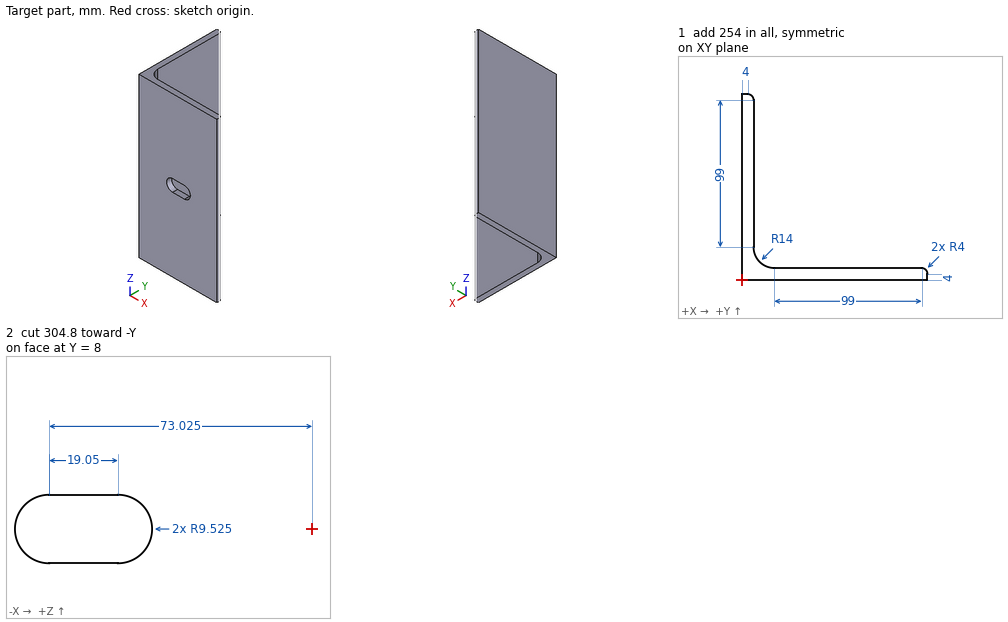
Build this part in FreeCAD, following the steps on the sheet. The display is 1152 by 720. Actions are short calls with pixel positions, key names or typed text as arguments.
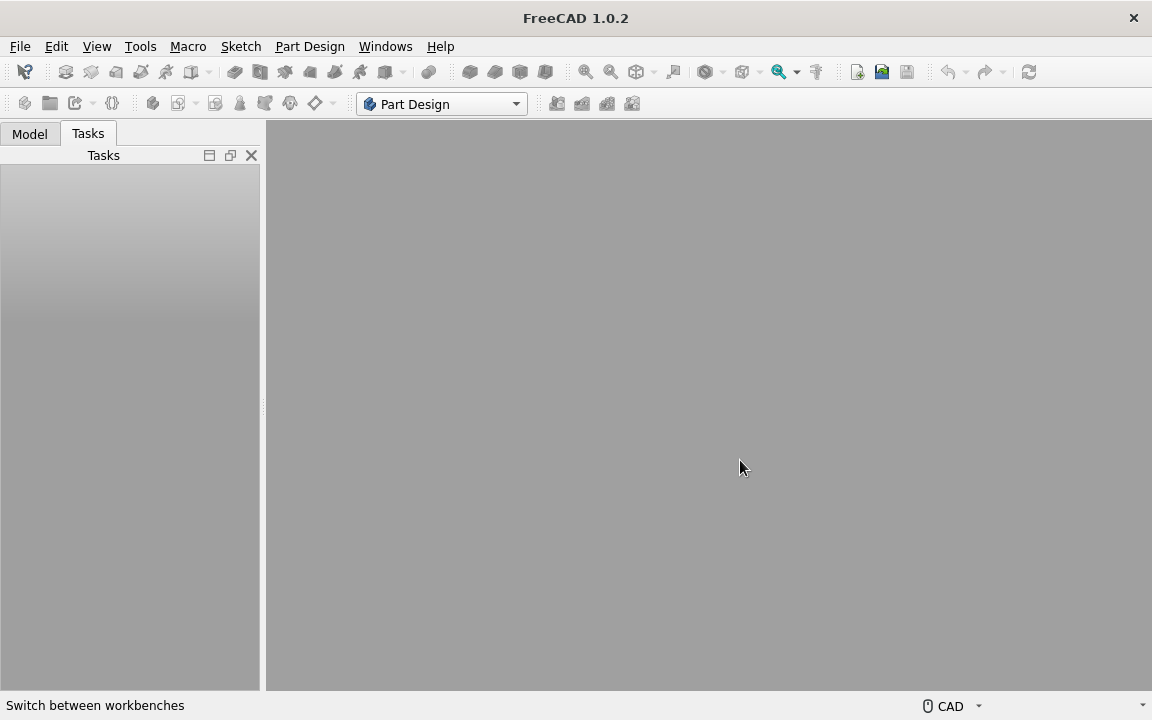
key(ctrl+n)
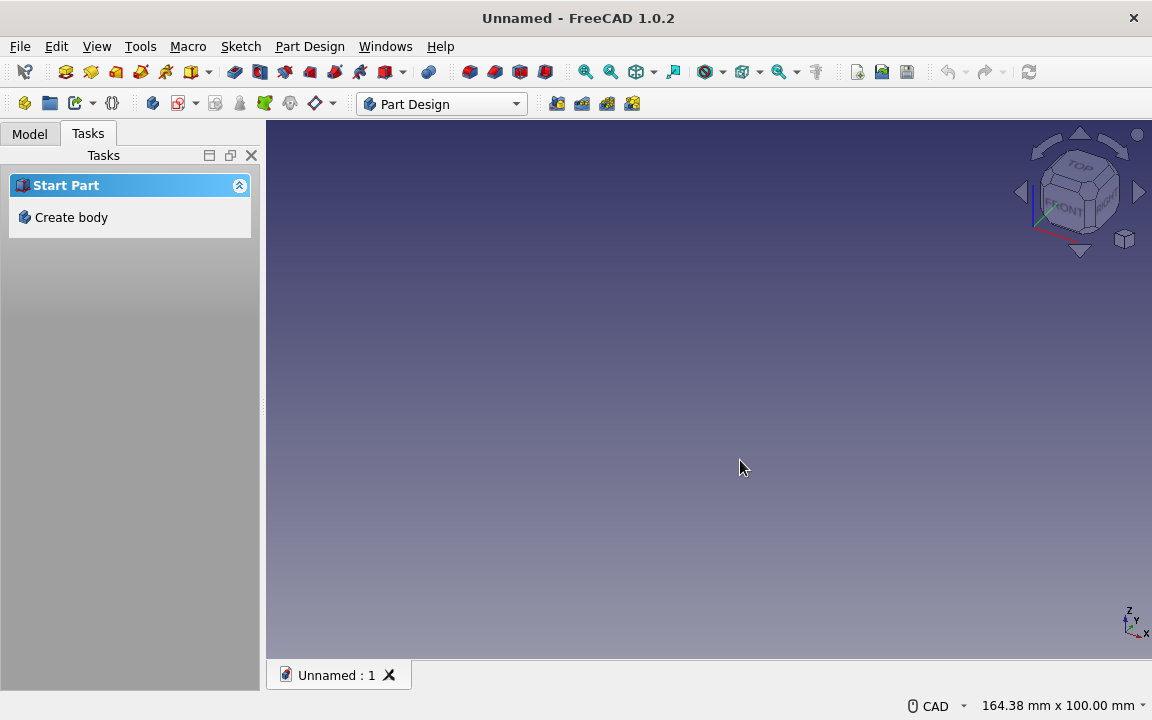
click(178, 104)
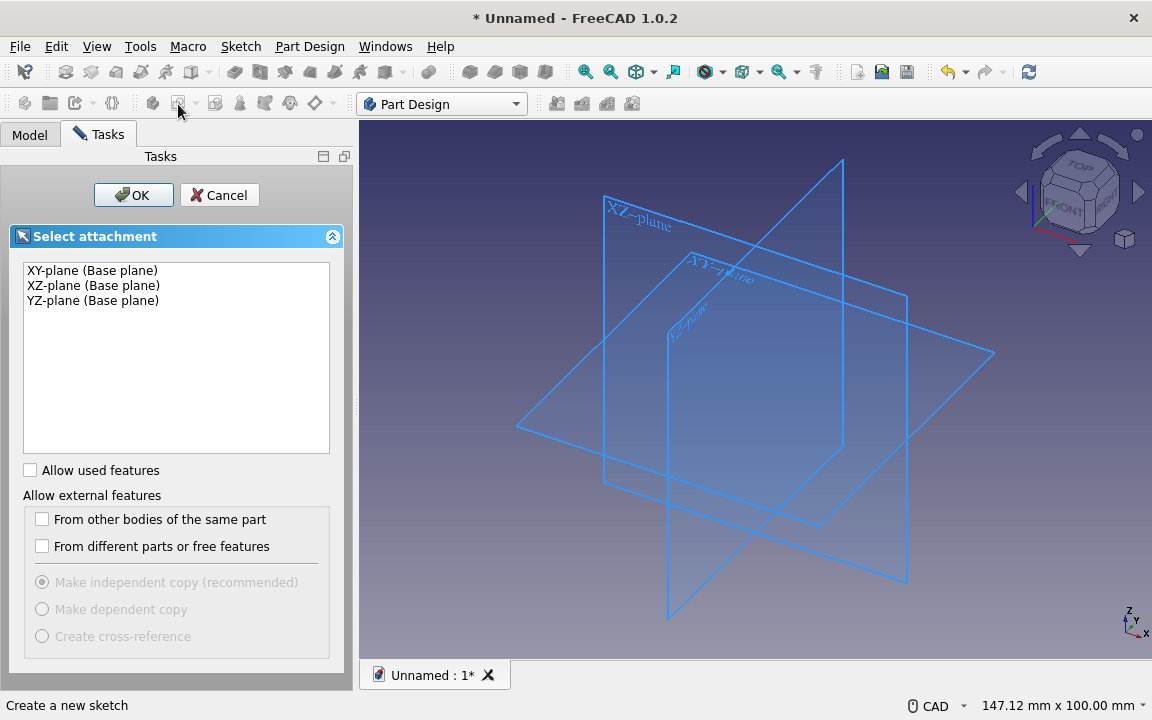
click(84, 270)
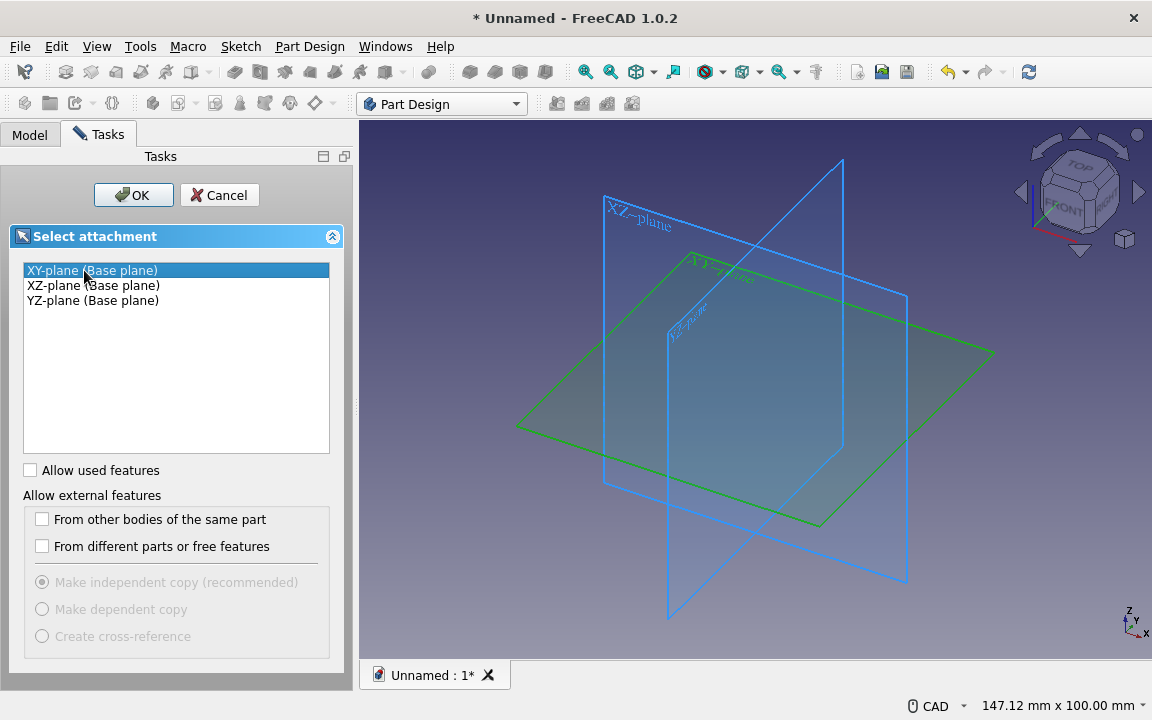
click(134, 195)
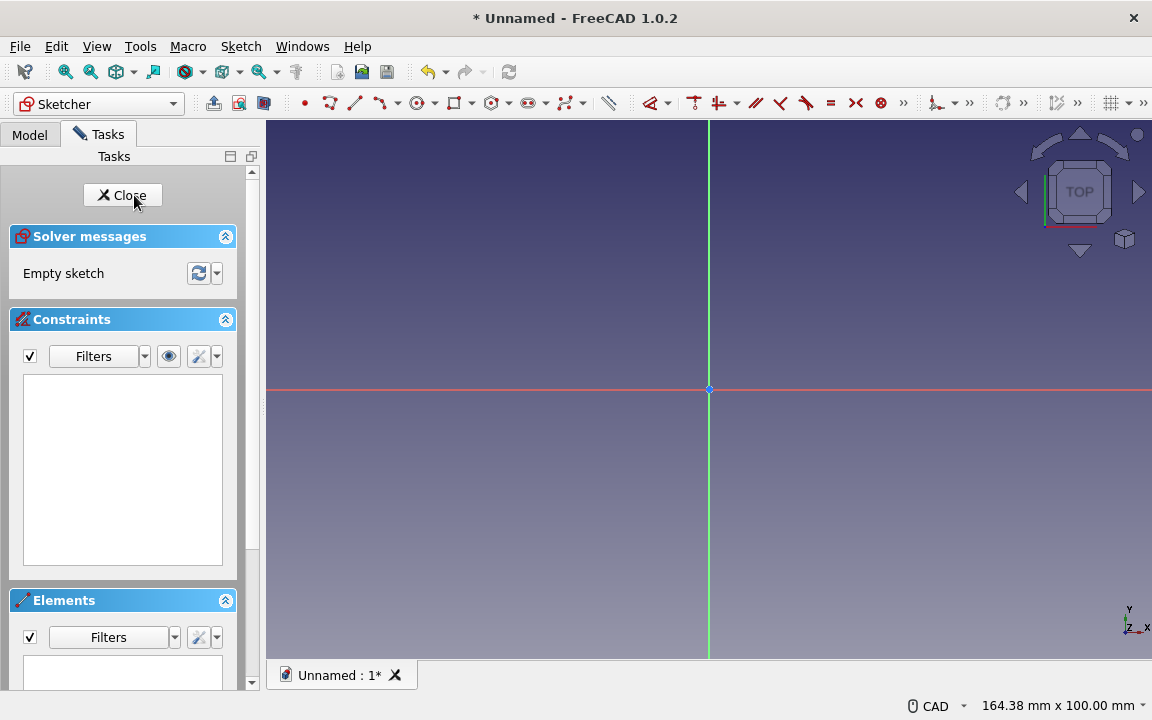
scroll(310, 631, down, 4)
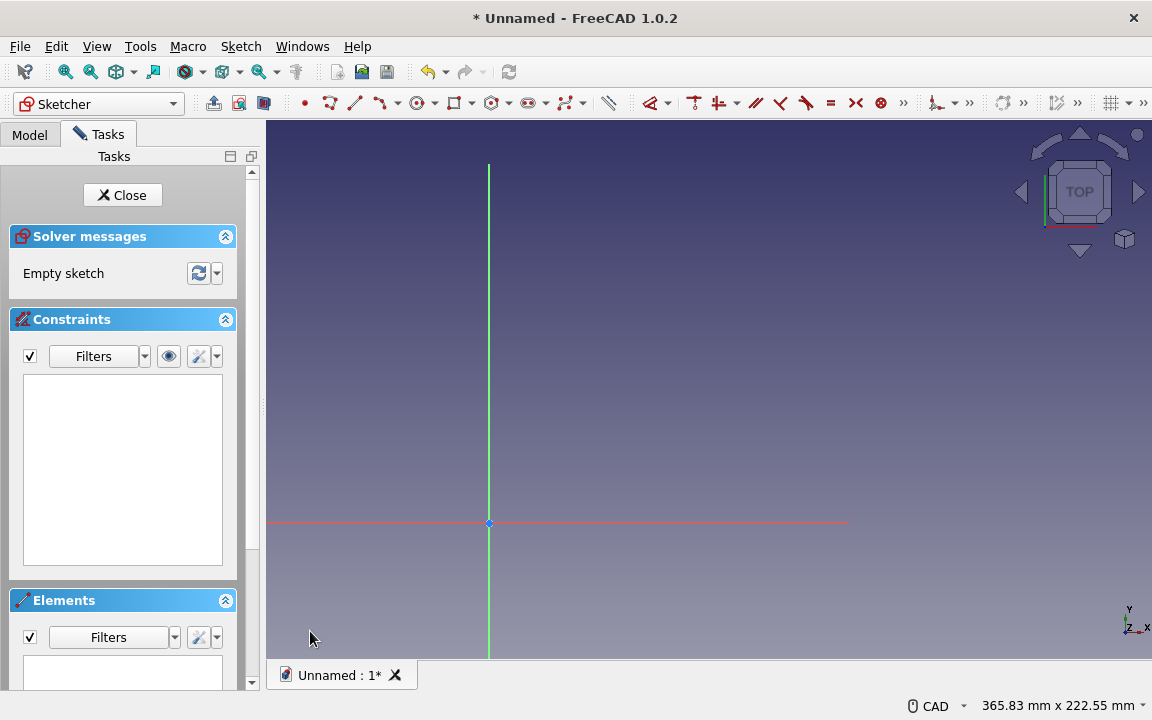
click(355, 104)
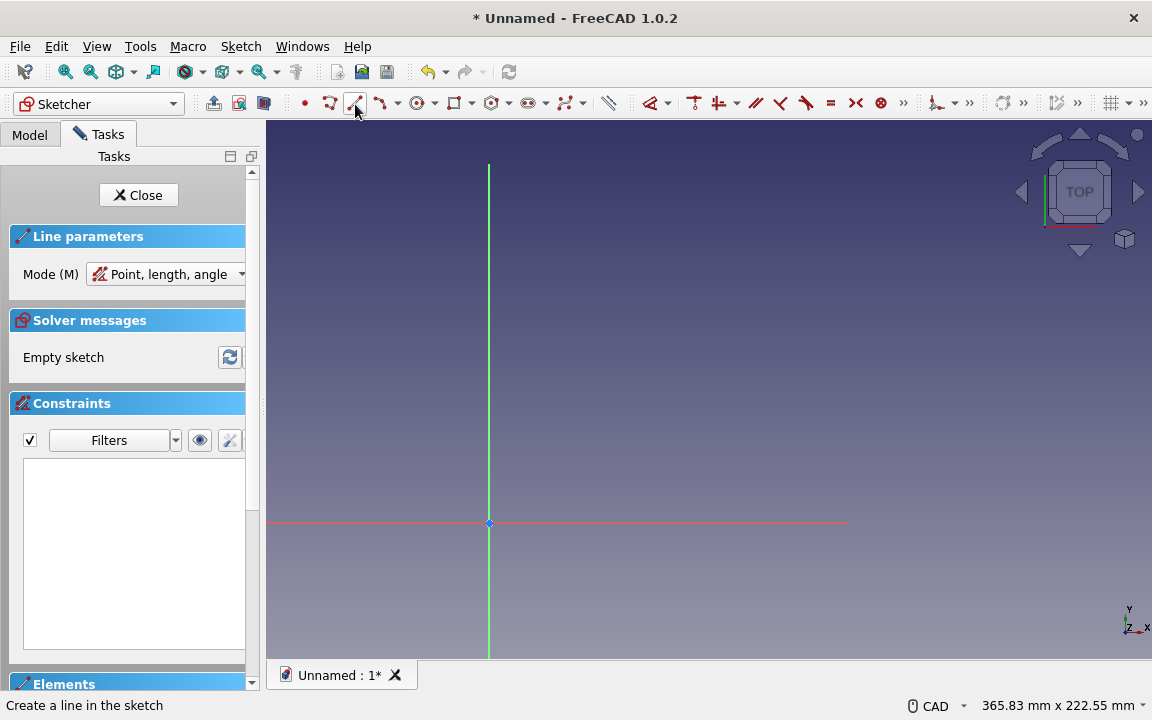
click(782, 504)
click(543, 504)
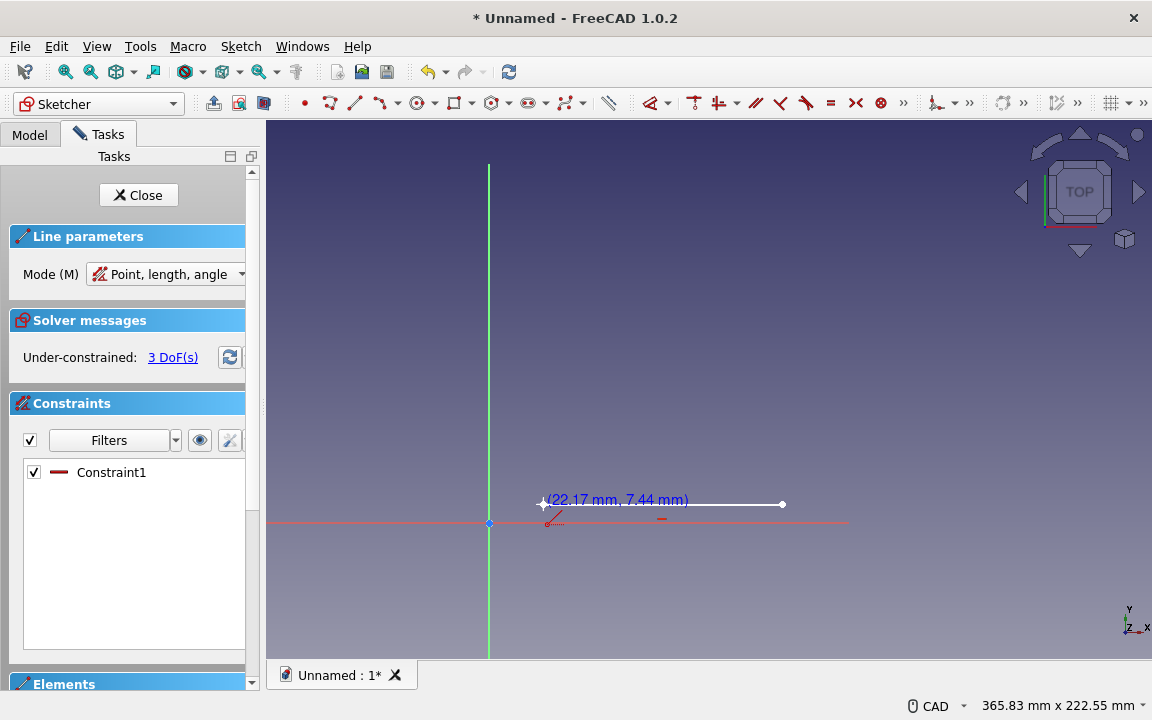
click(509, 470)
click(509, 230)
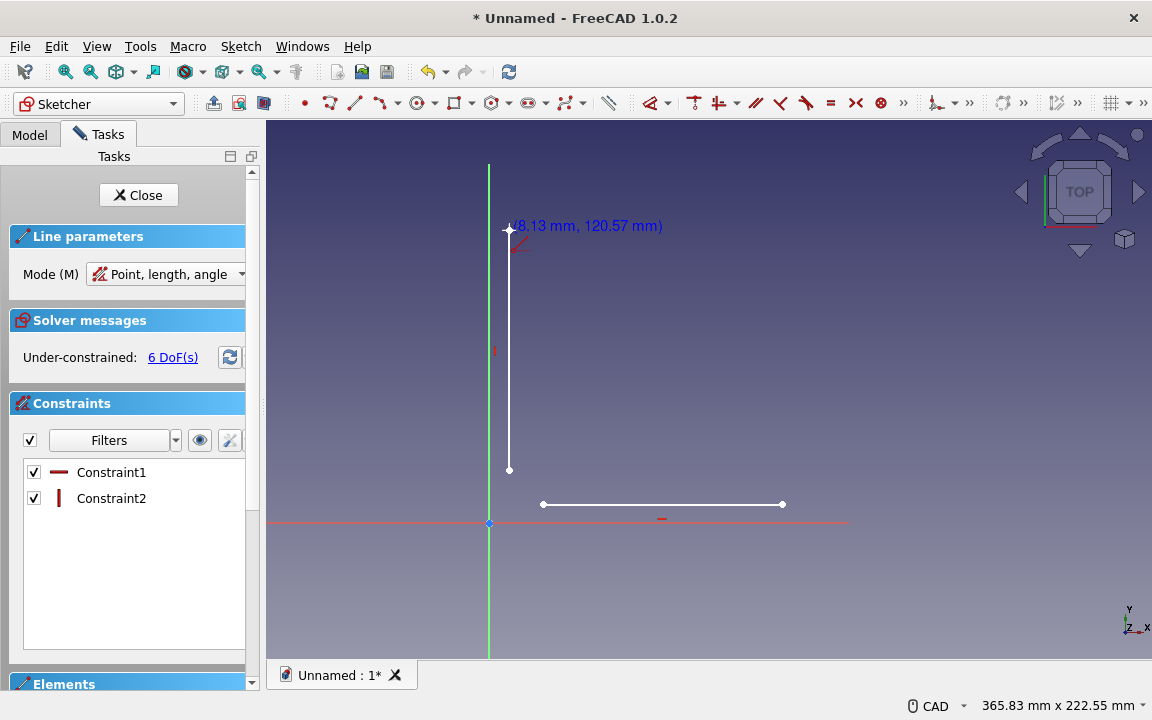
click(330, 104)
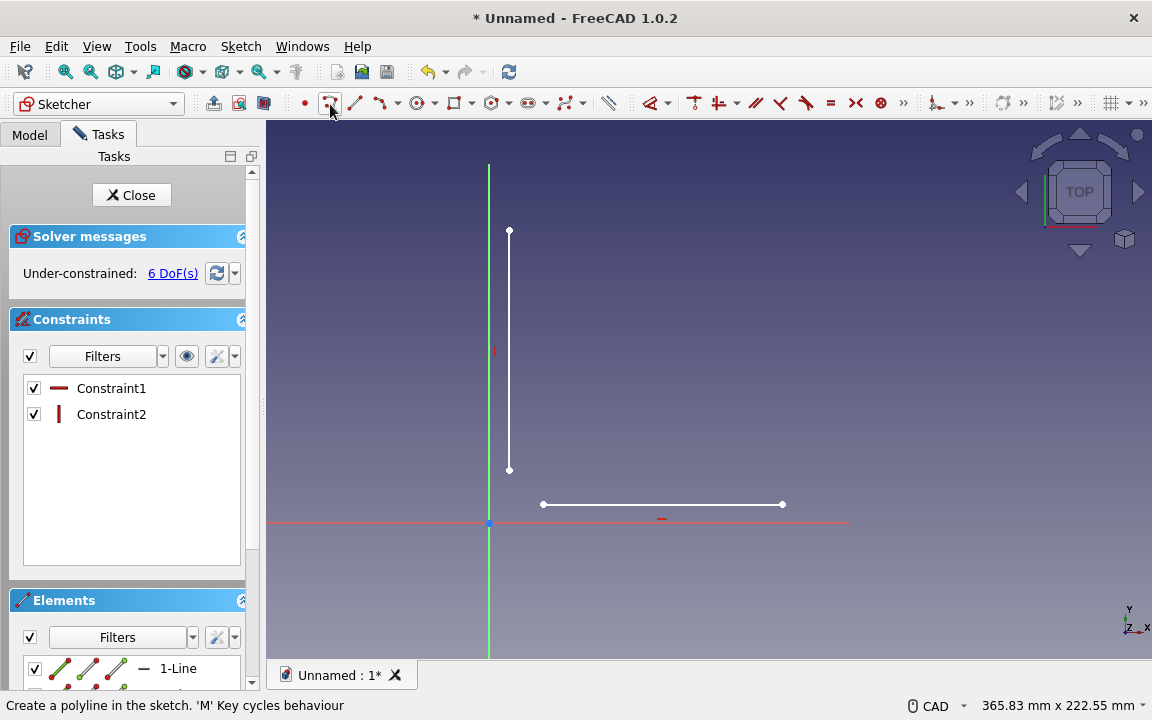
scroll(499, 220, up, 3)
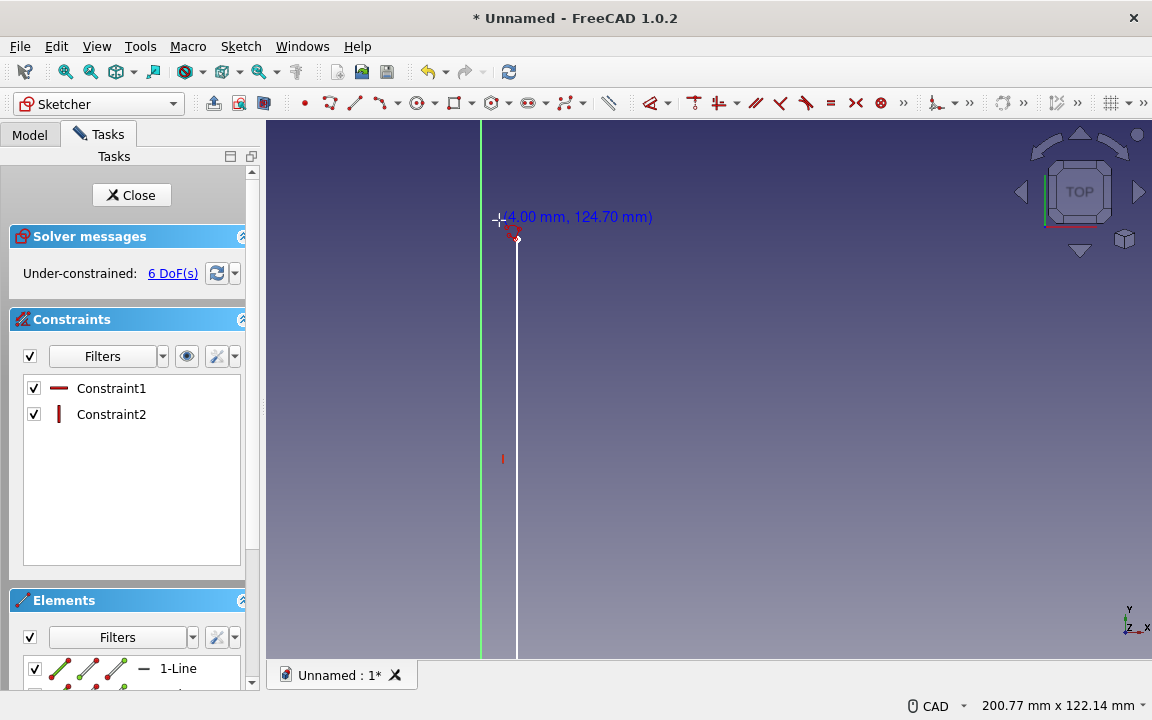
click(499, 220)
click(481, 220)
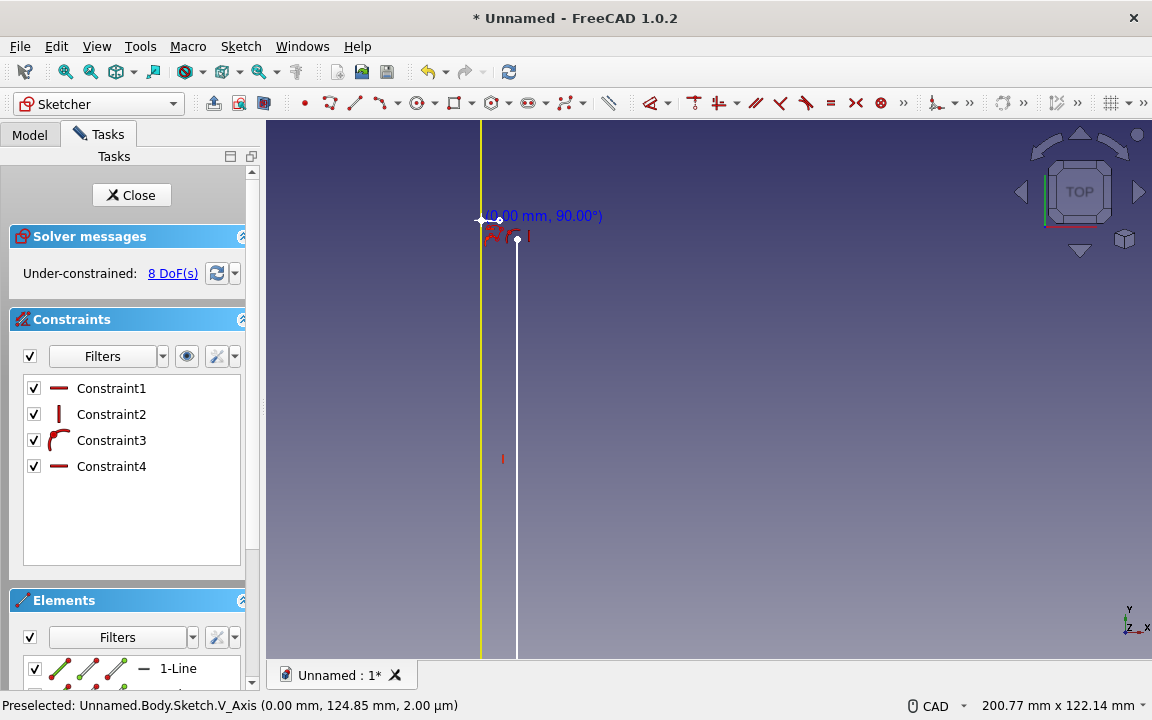
scroll(404, 173, down, 2)